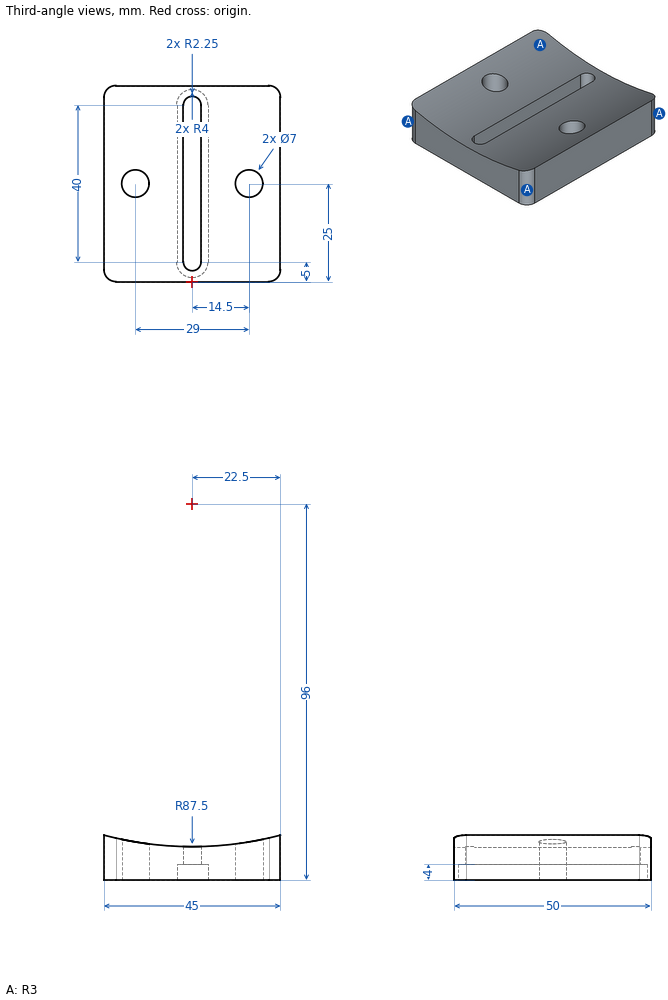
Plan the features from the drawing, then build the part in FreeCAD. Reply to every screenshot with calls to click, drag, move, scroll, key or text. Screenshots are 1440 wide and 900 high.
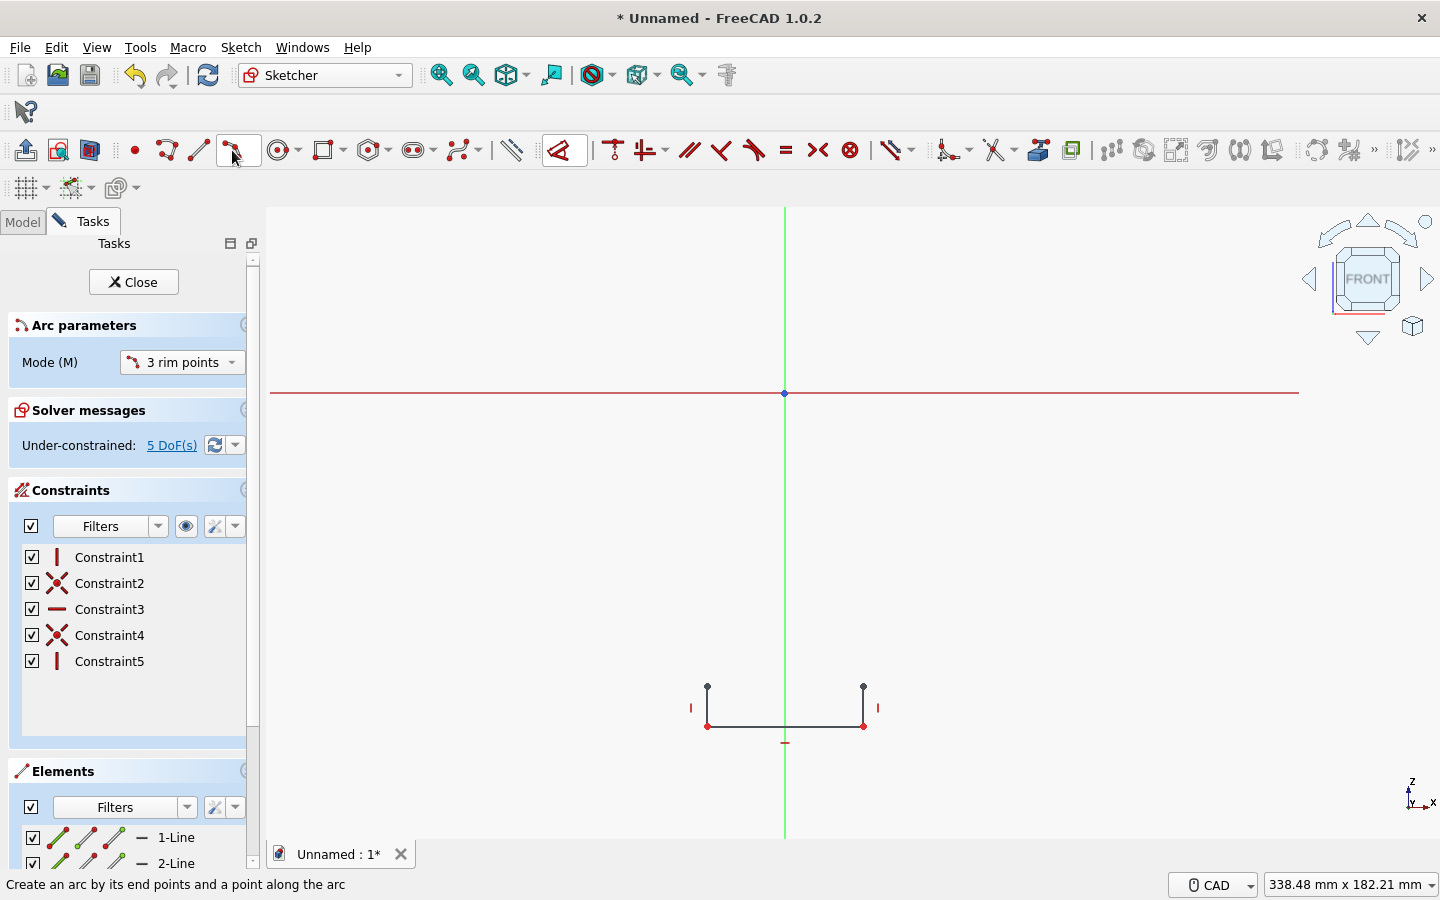
click(707, 687)
click(863, 687)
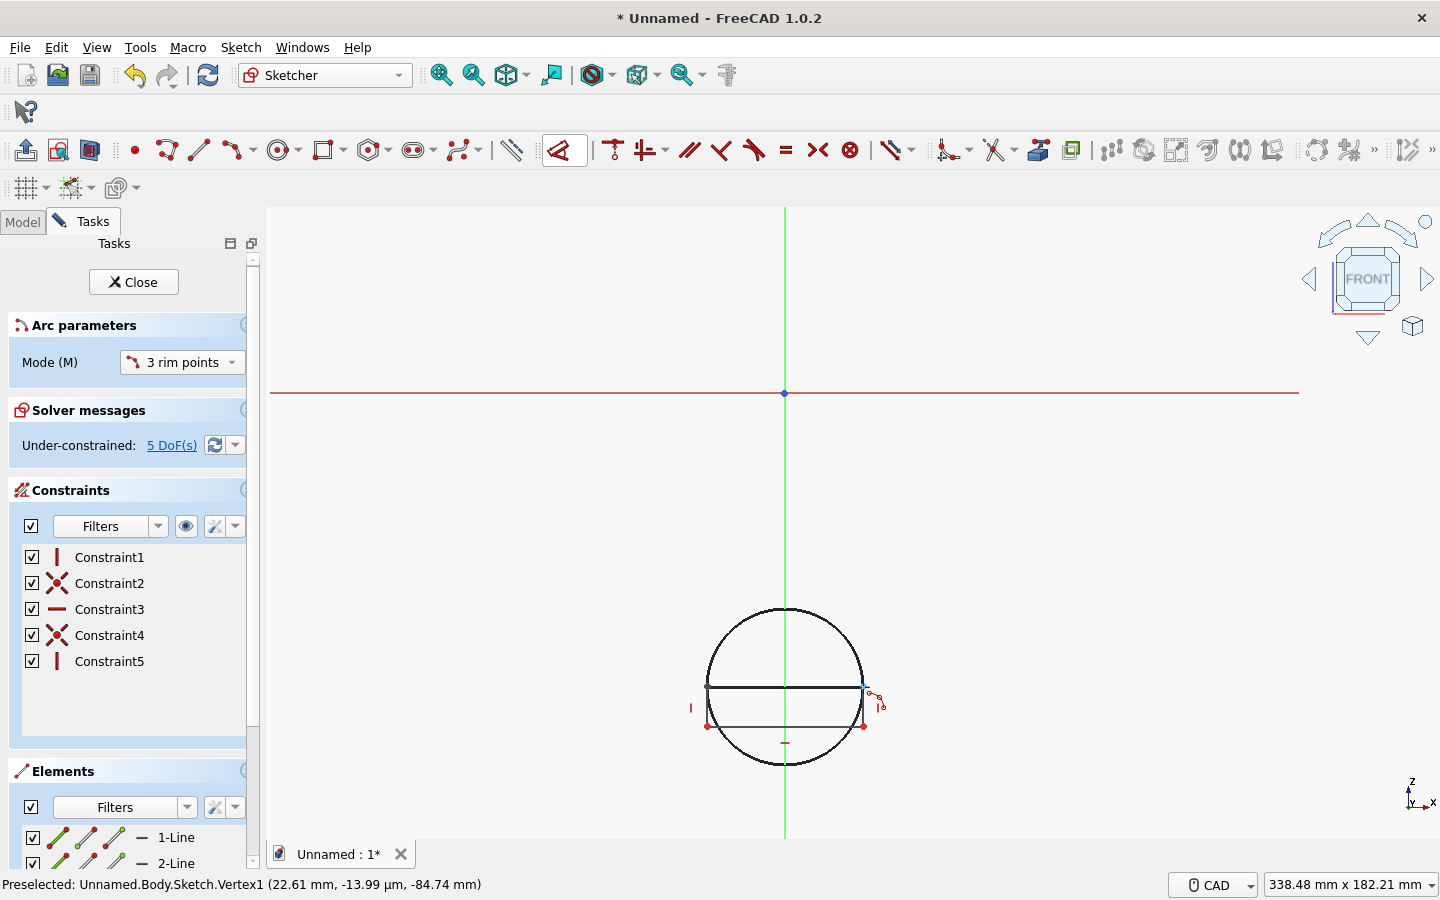
scroll(769, 696, up, 3)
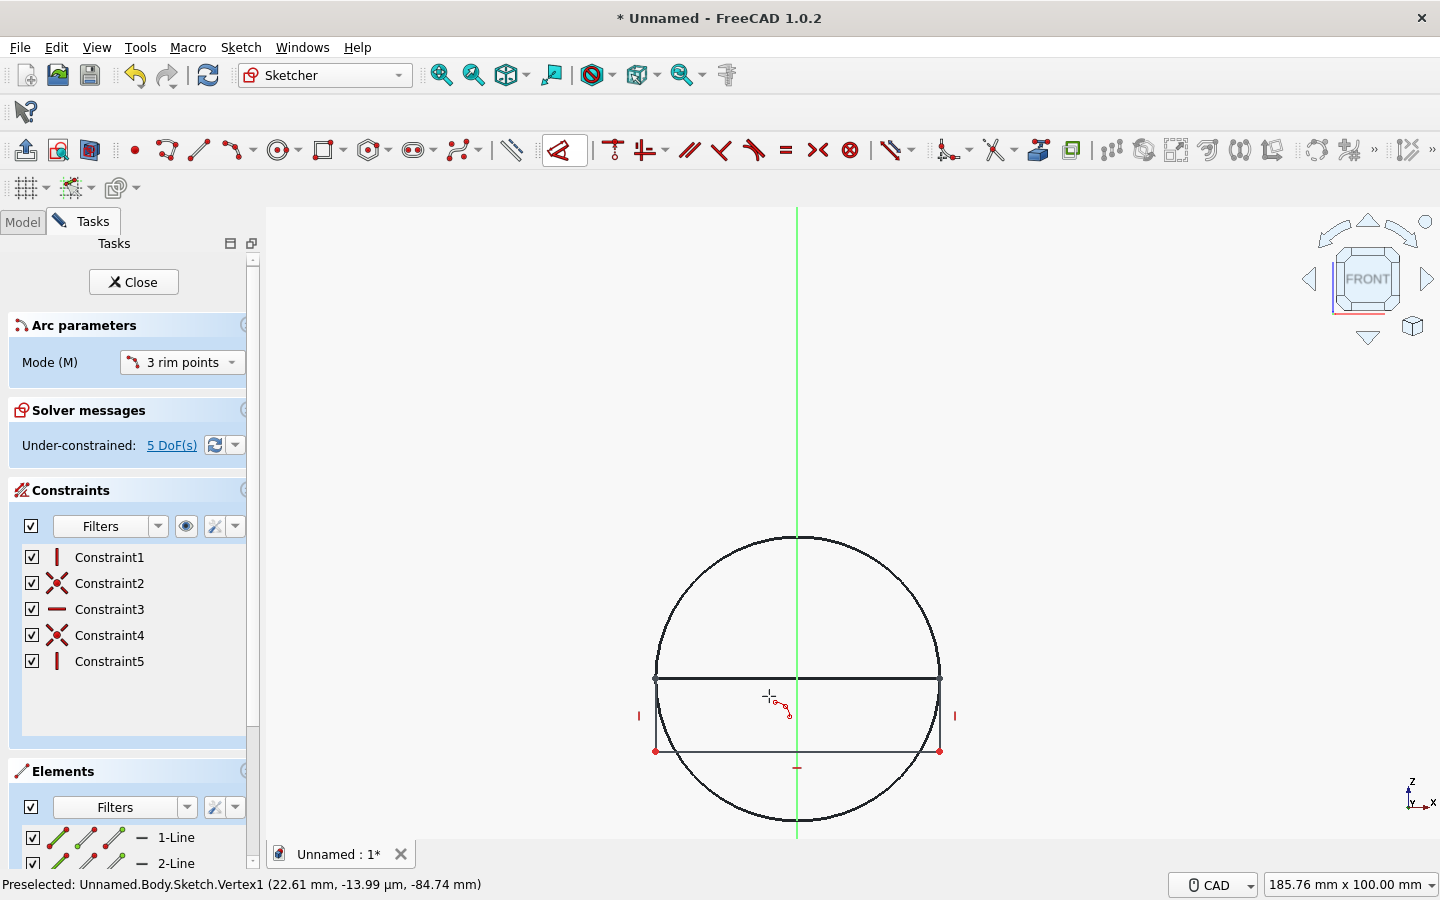
click(768, 696)
key(Escape)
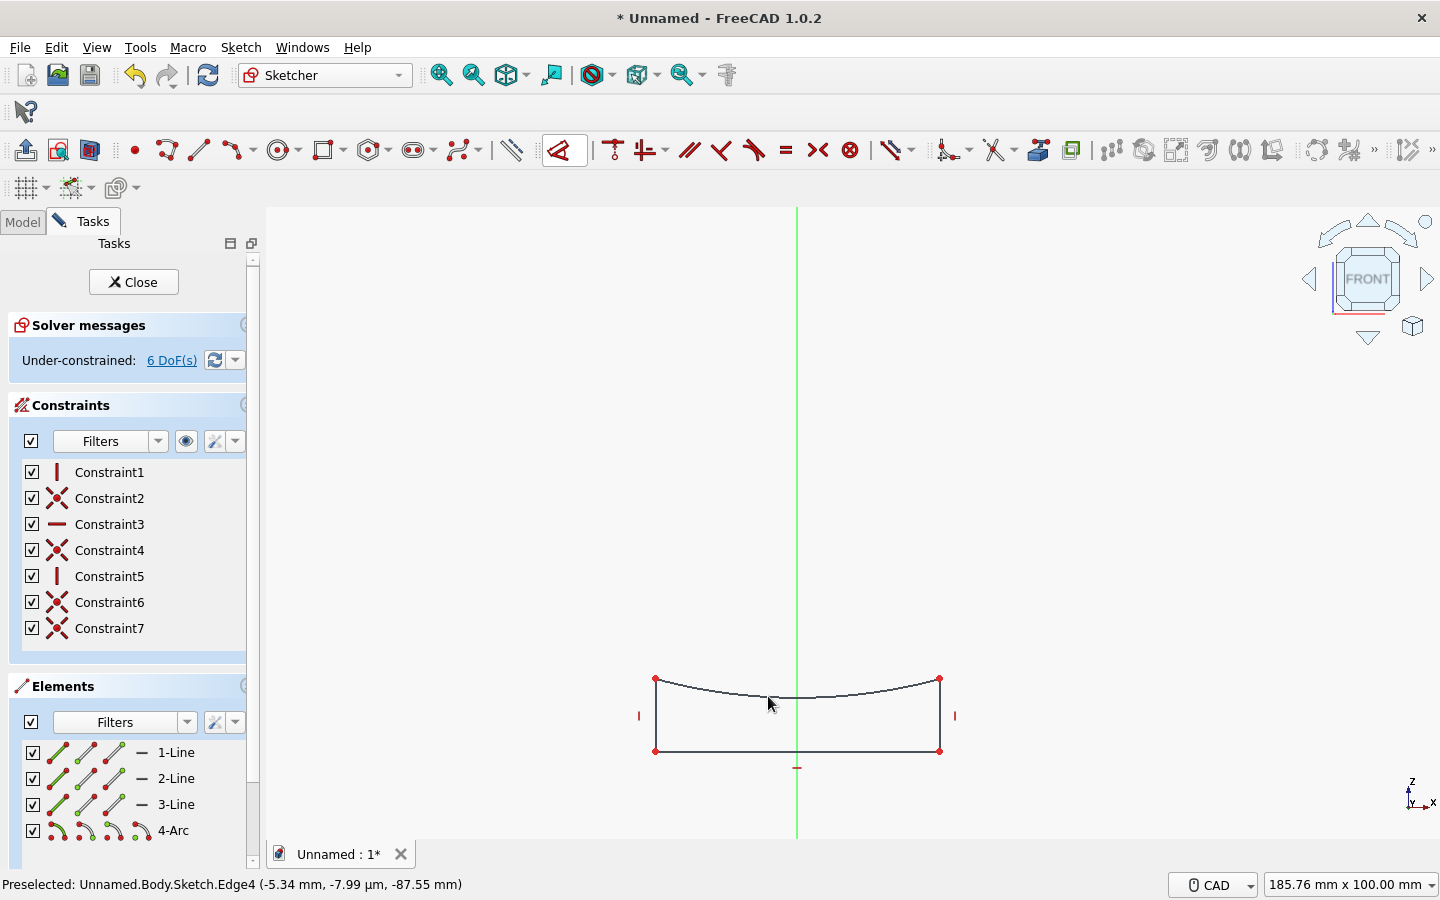
scroll(759, 678, down, 2)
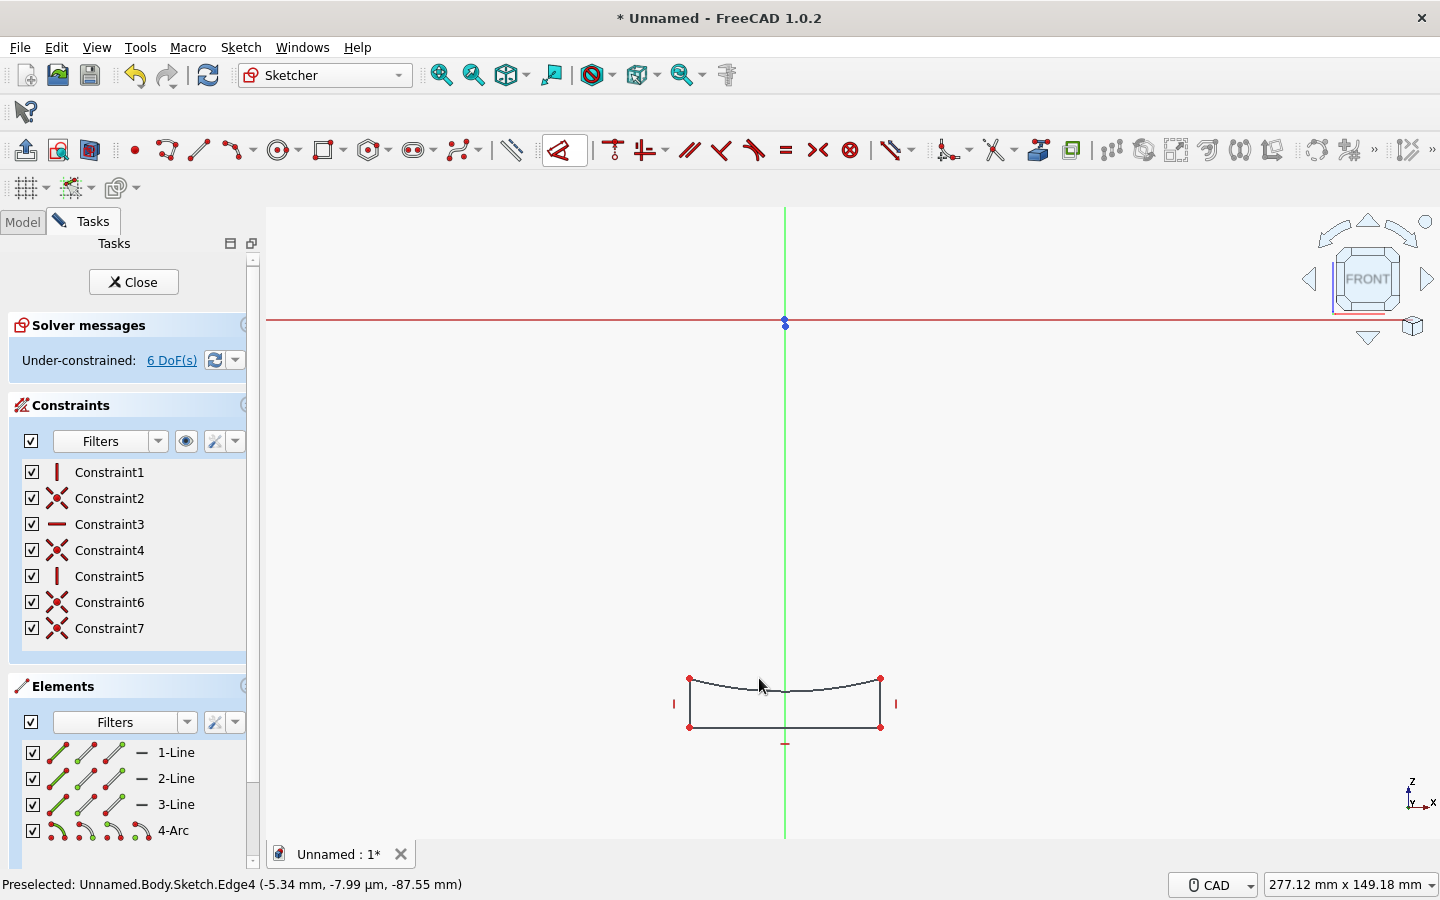
drag(775, 310, 795, 336)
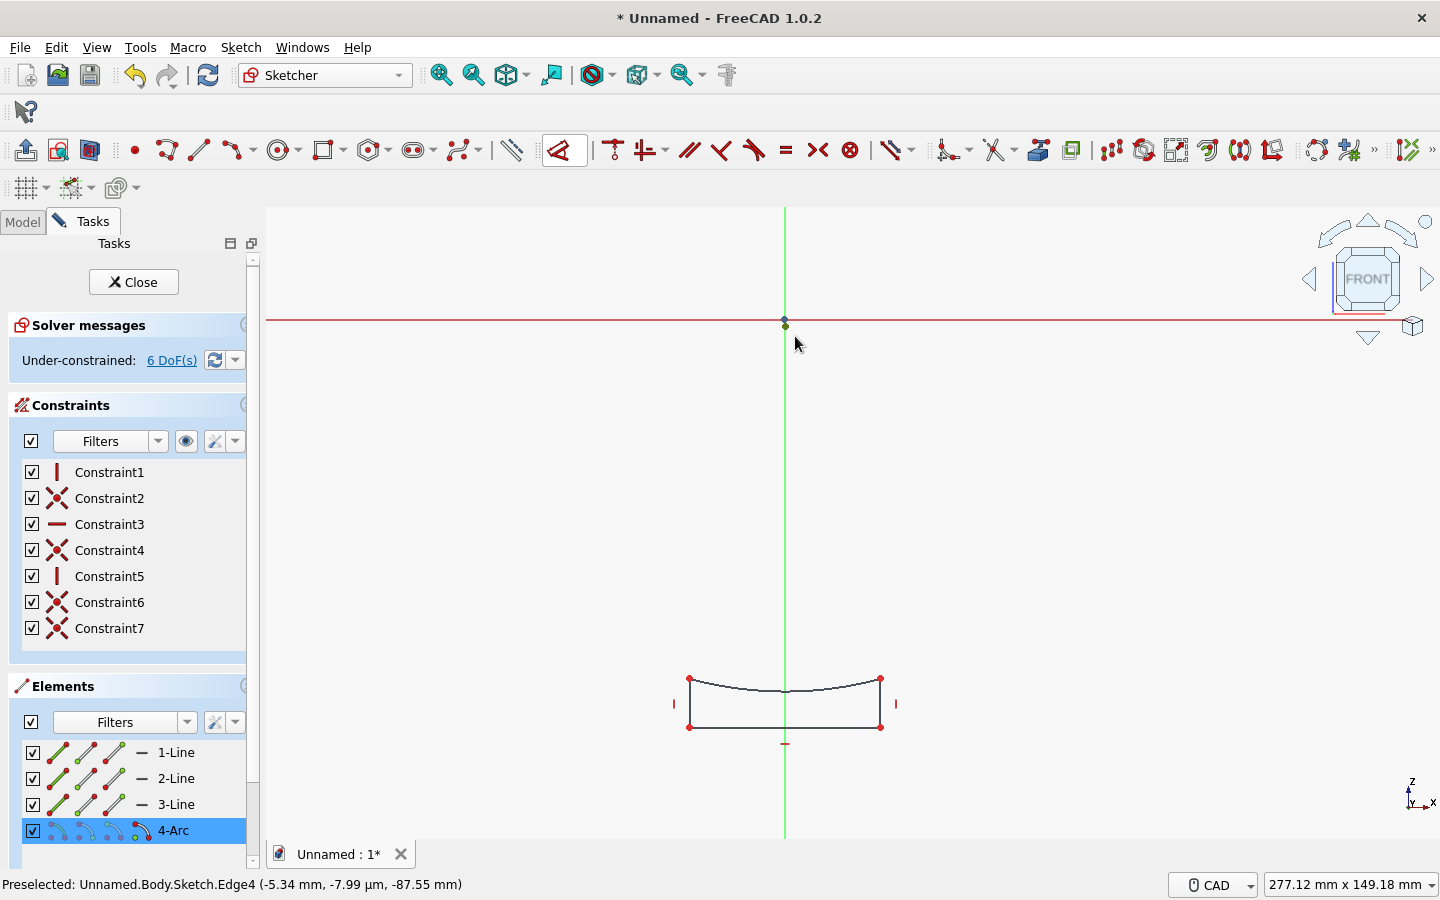
click(614, 150)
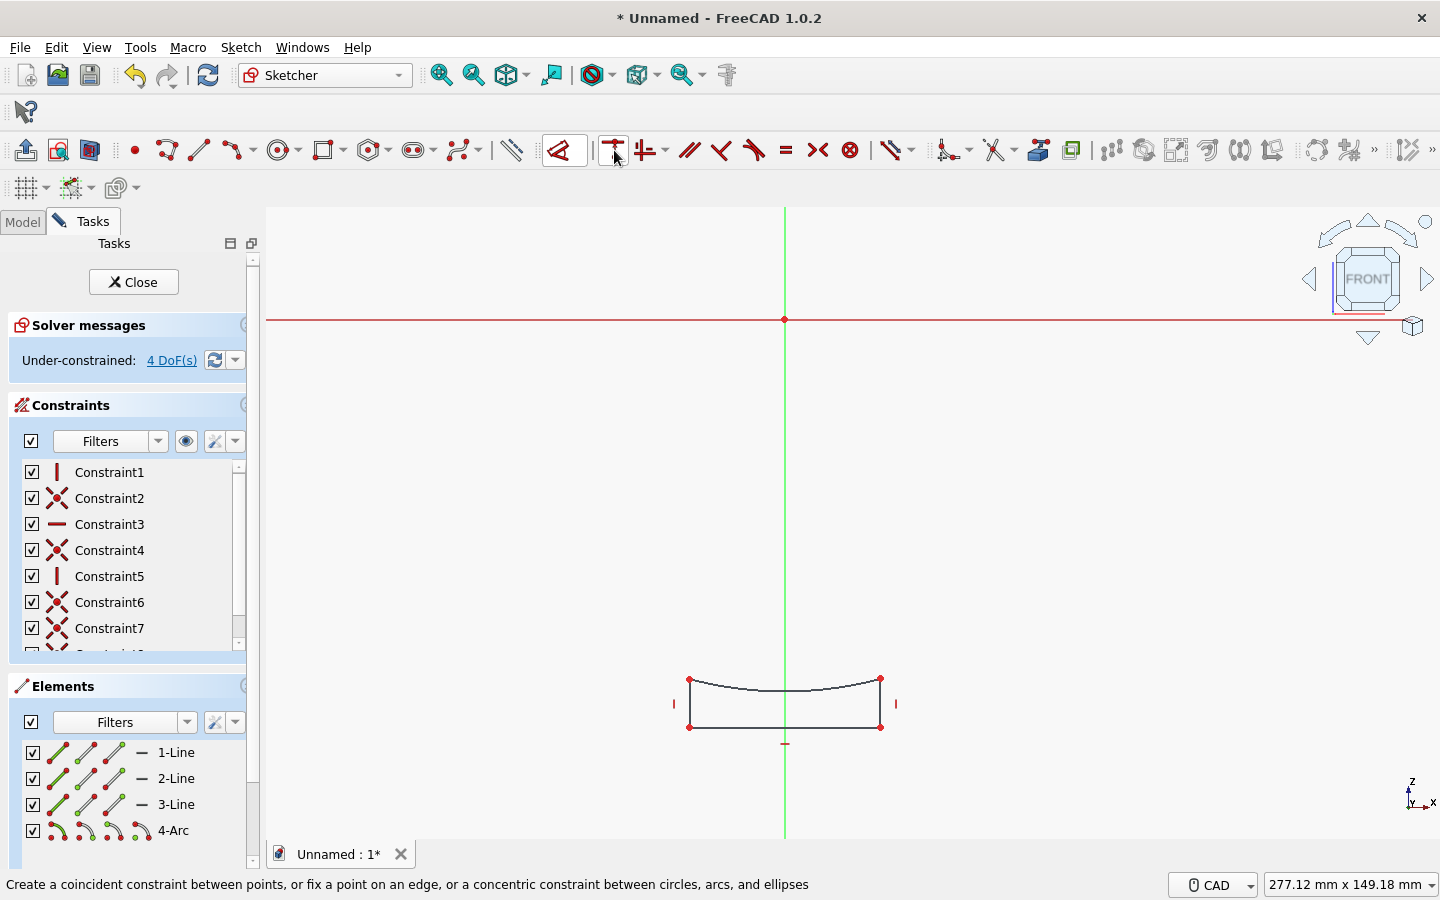
key(d)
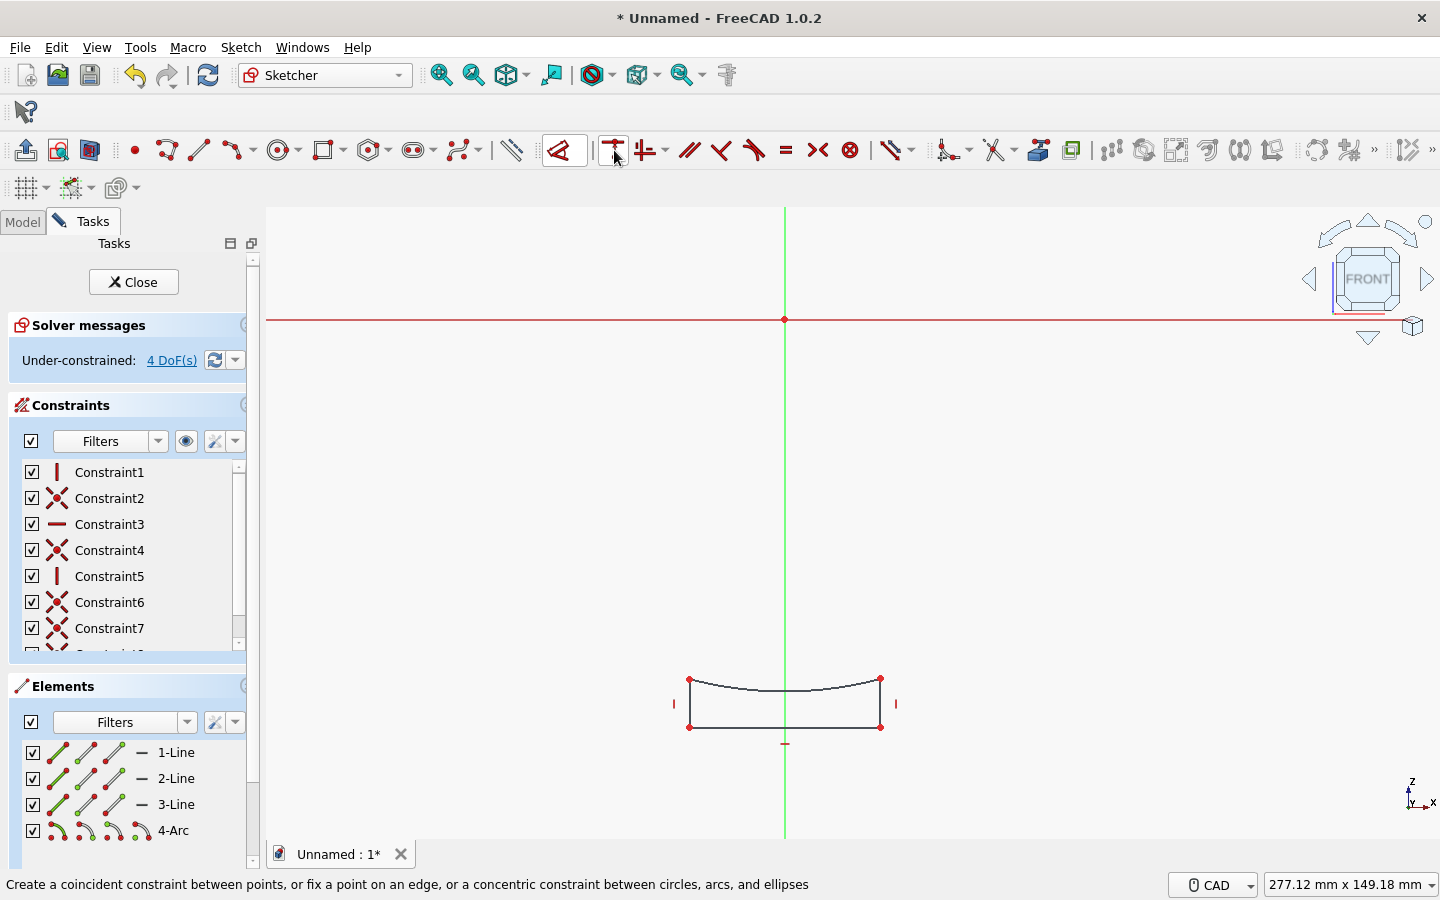
click(747, 690)
click(556, 653)